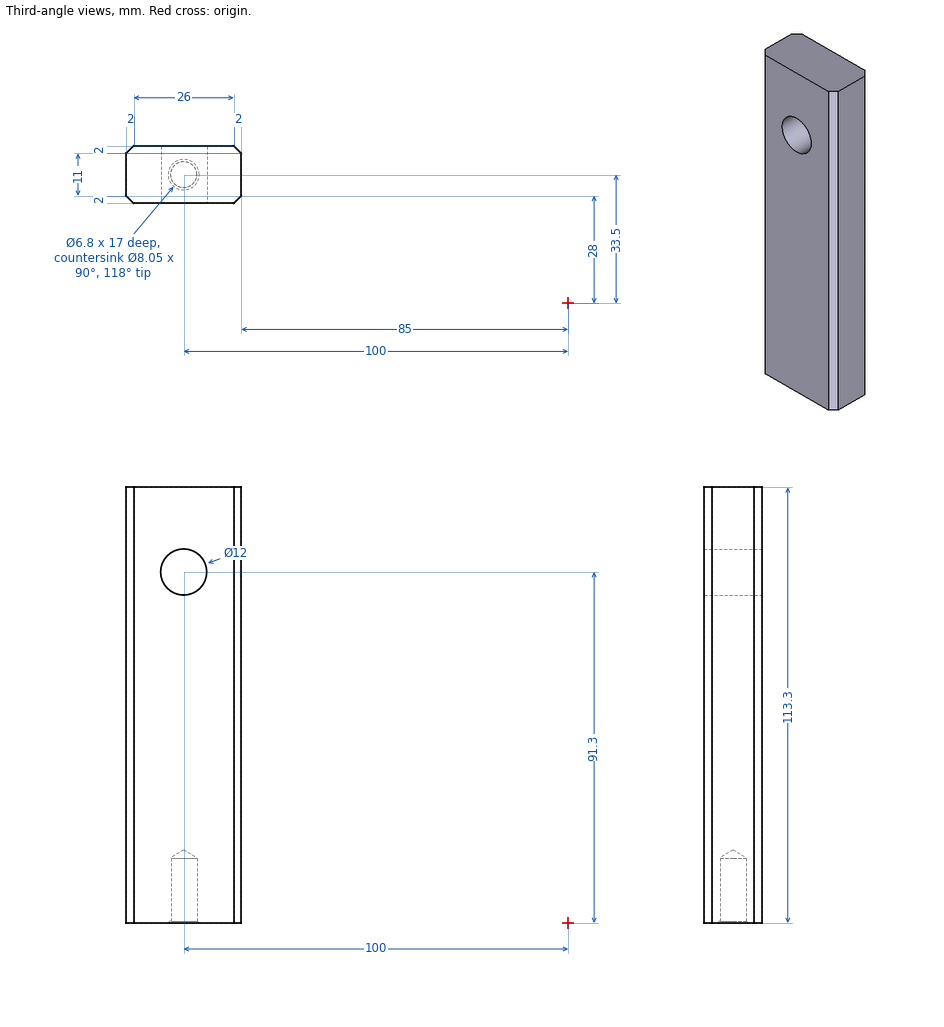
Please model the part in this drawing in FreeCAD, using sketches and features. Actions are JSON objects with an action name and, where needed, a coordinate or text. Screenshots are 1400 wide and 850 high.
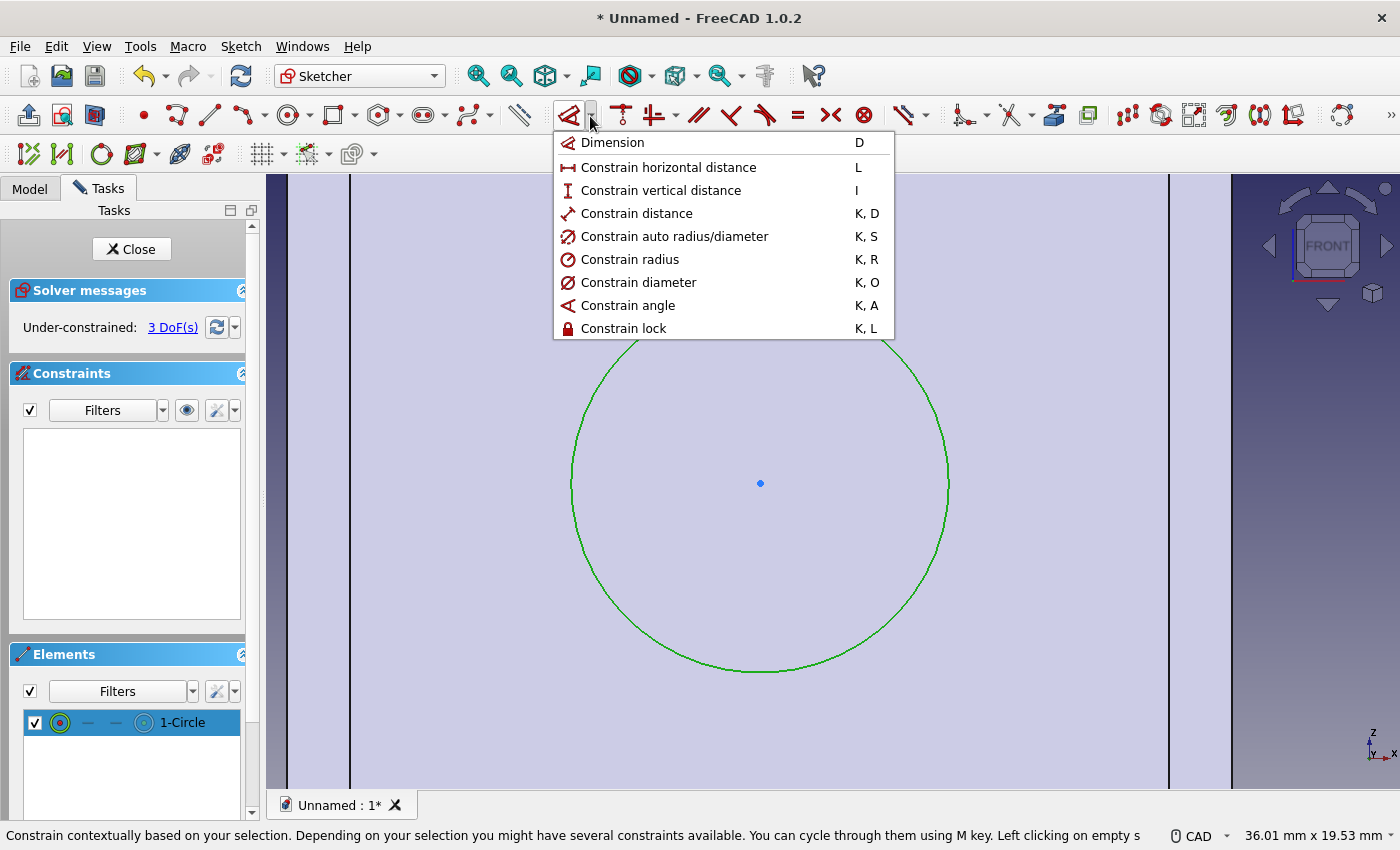
{"action": "left_click", "coordinate": [724, 282]}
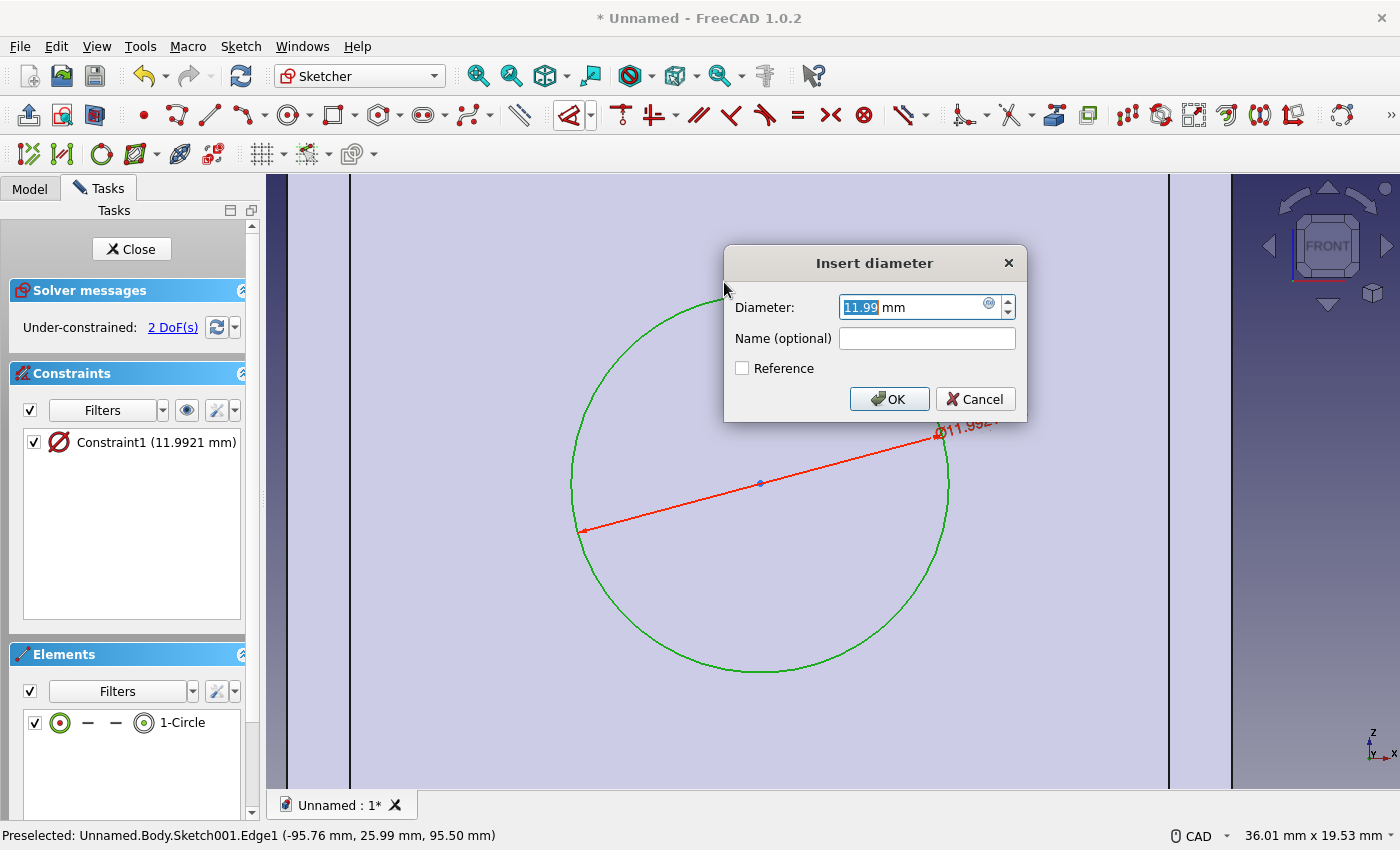
{"action": "type", "text": "12"}
{"action": "key", "text": "Return"}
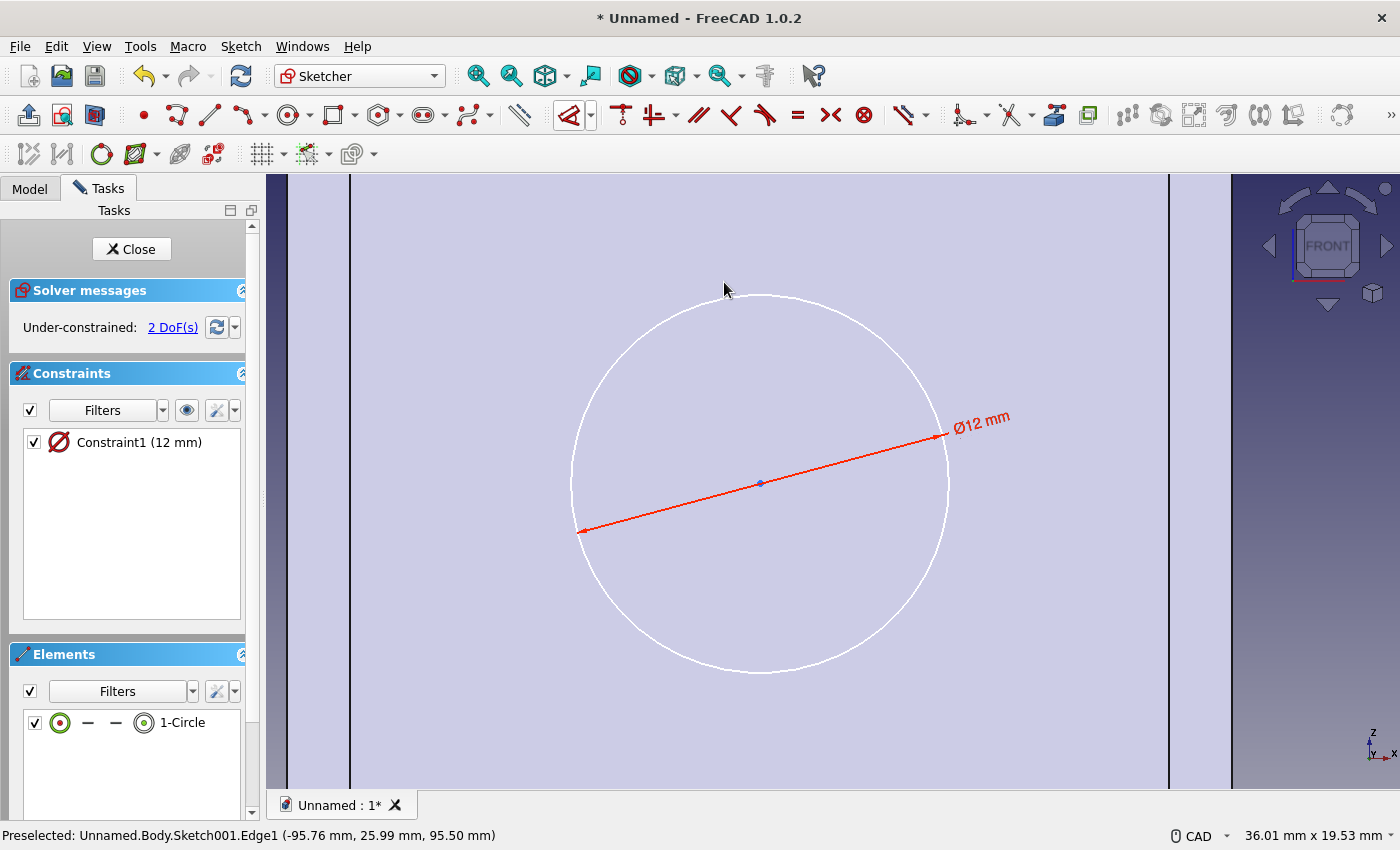
{"action": "left_click", "coordinate": [760, 484]}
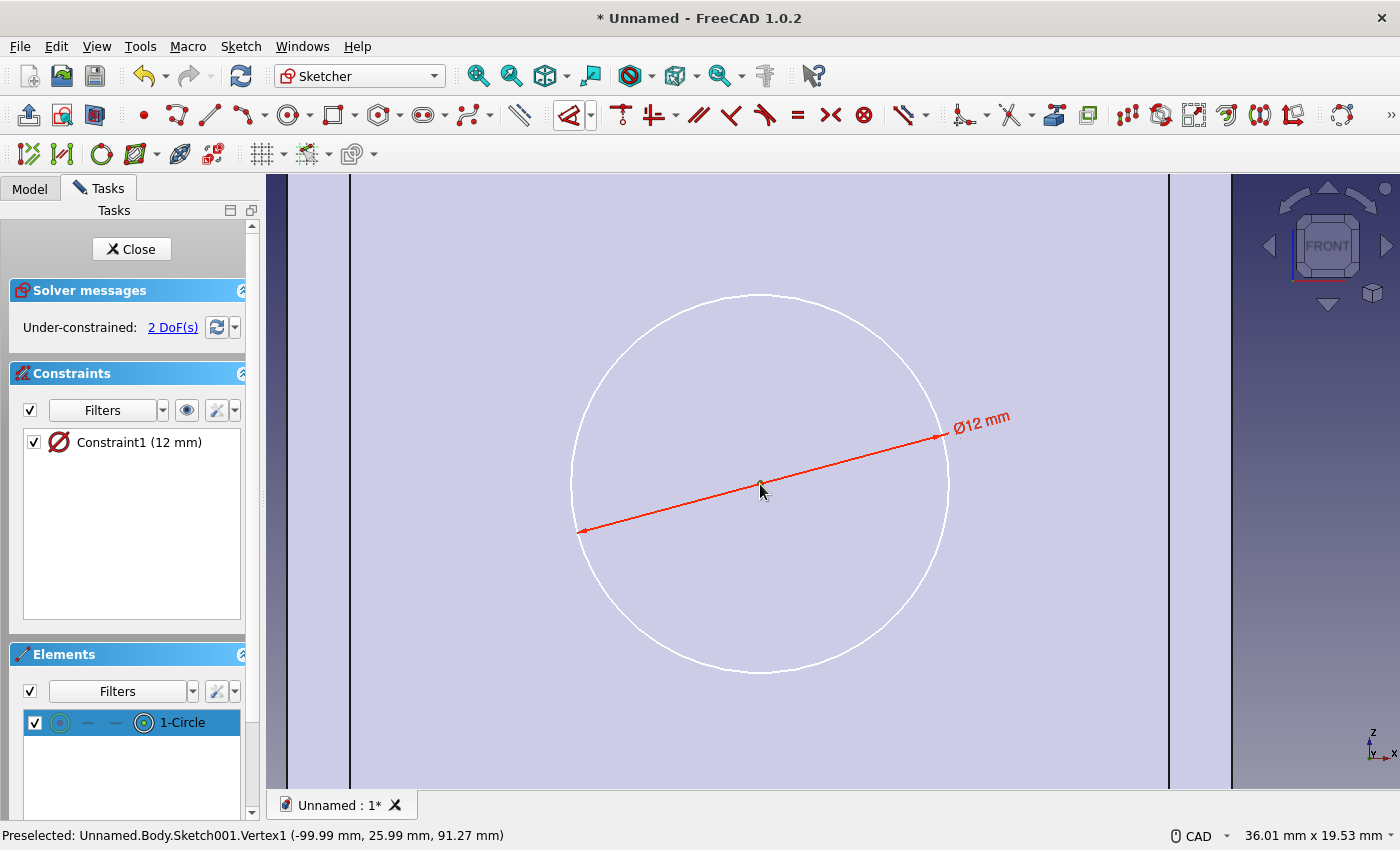
{"action": "left_click", "coordinate": [590, 116]}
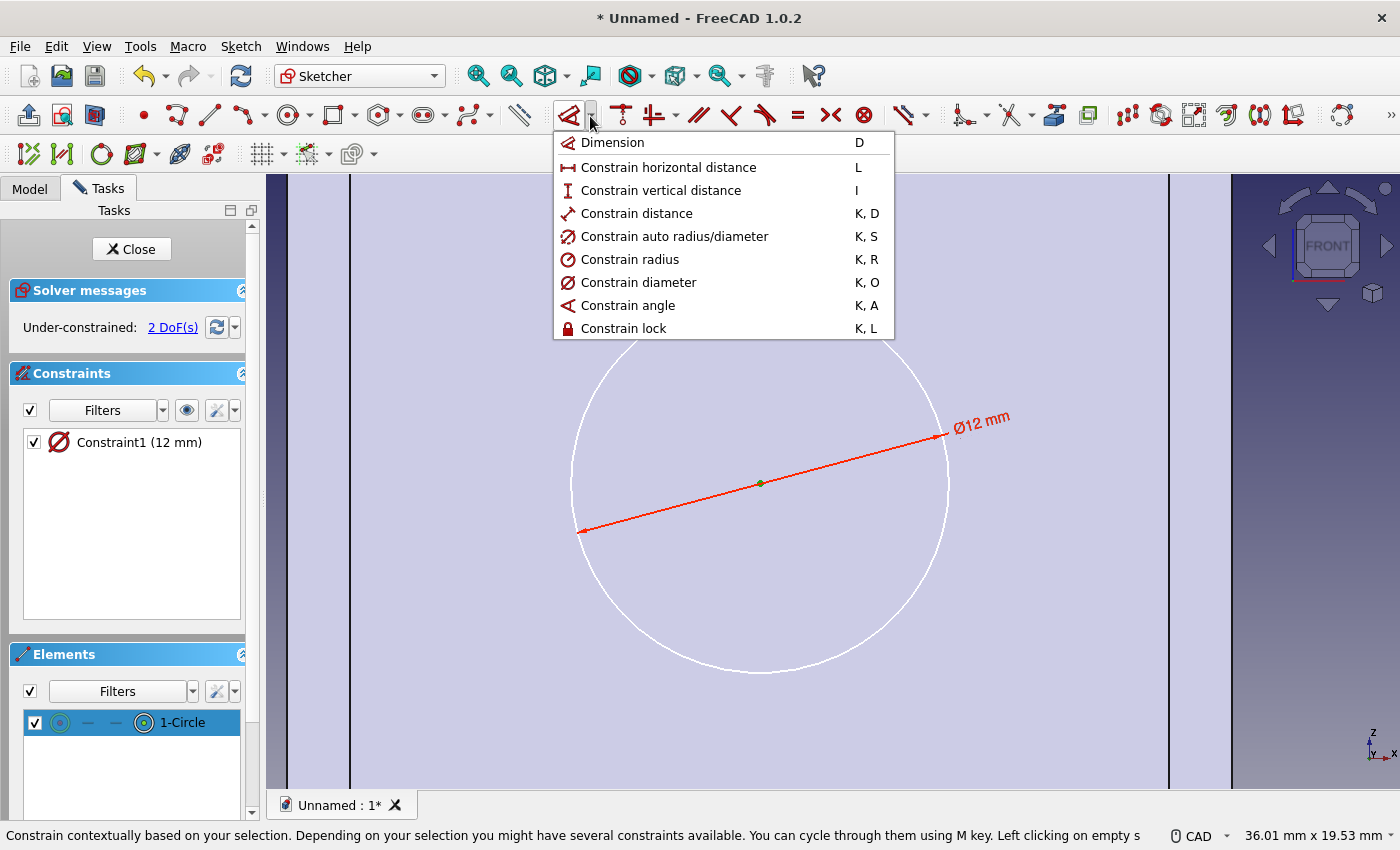
{"action": "left_click", "coordinate": [724, 168]}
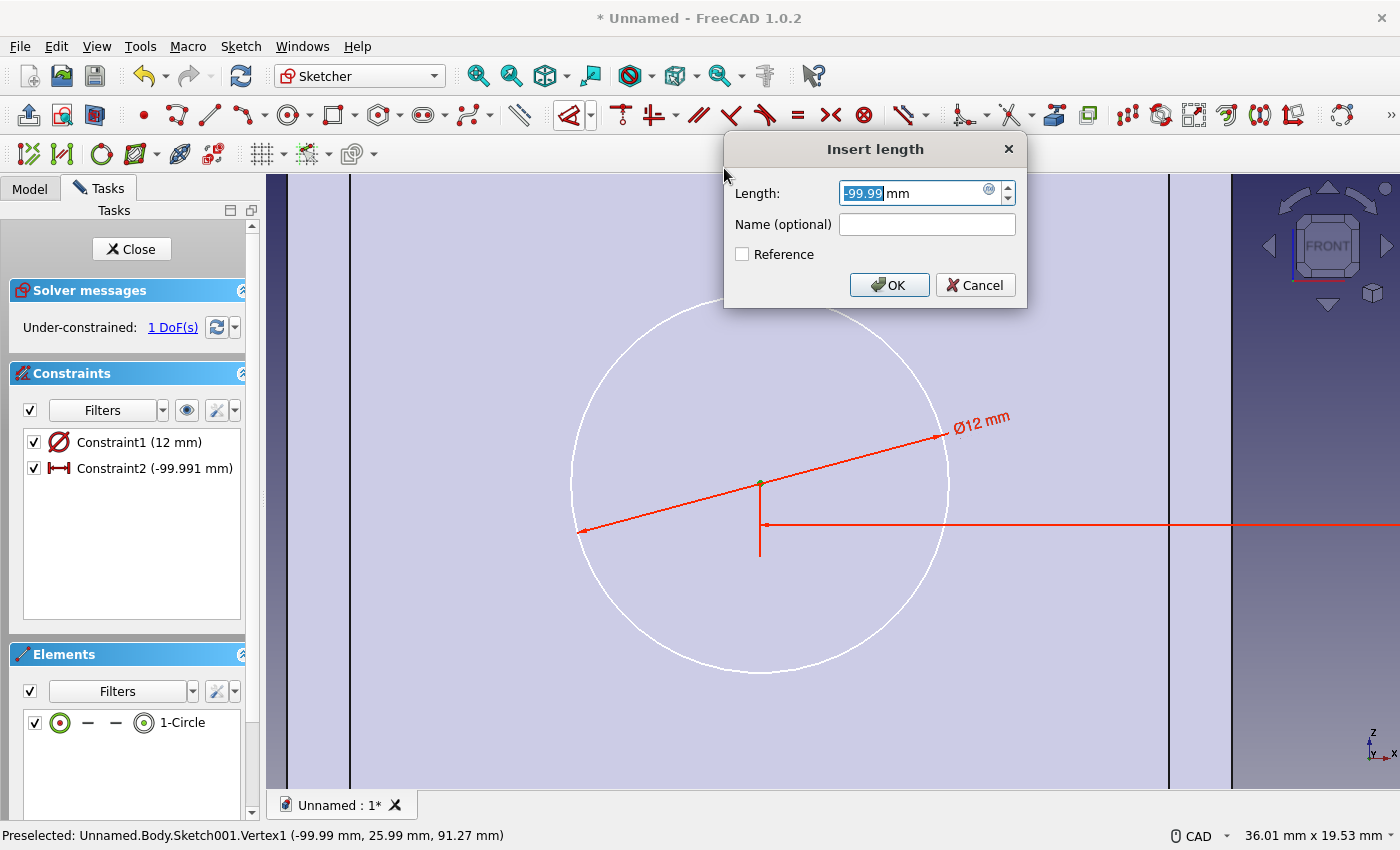
{"action": "type", "text": "-100"}
{"action": "key", "text": "Return"}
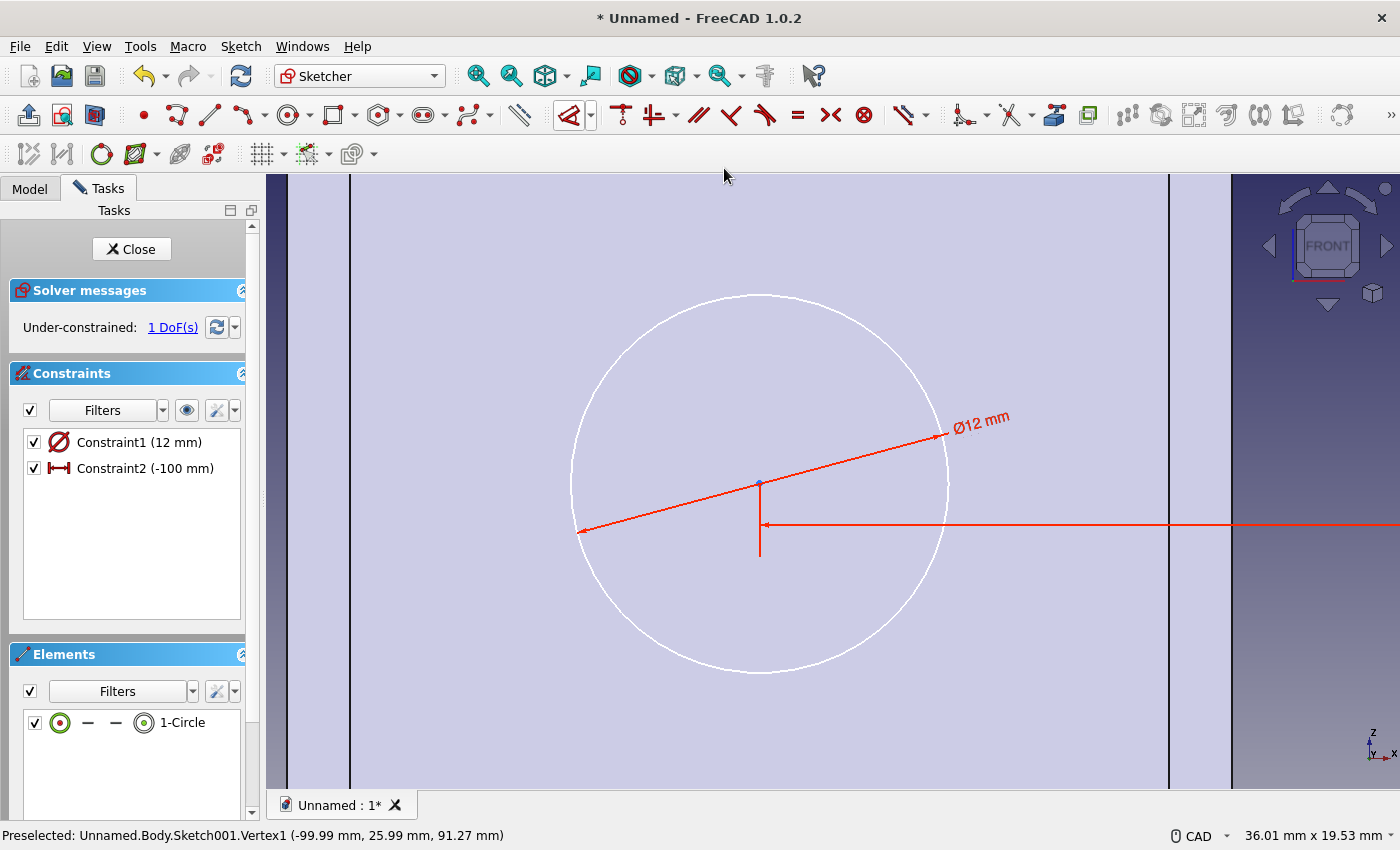
{"action": "left_click", "coordinate": [760, 484]}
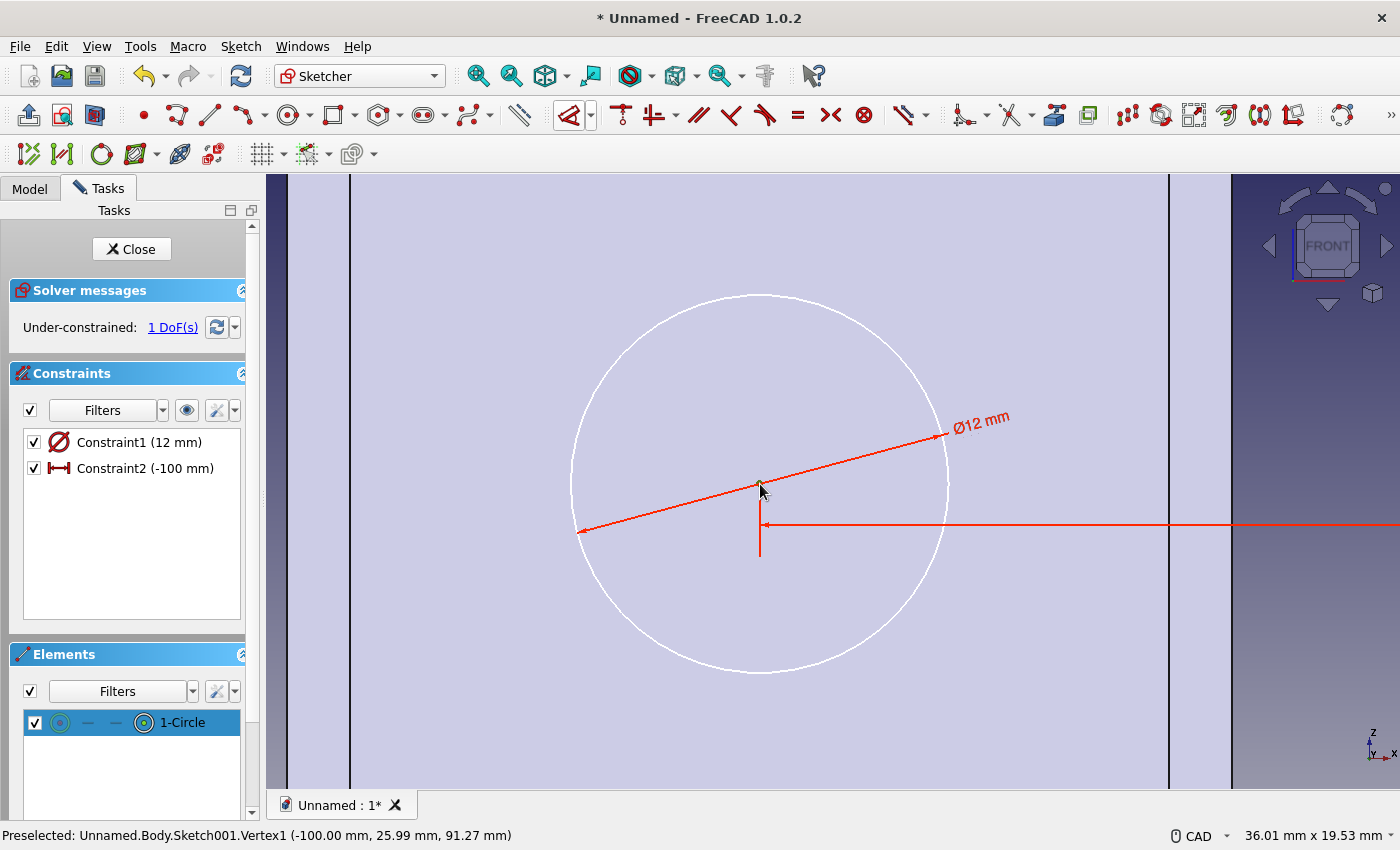
{"action": "key", "text": "i"}